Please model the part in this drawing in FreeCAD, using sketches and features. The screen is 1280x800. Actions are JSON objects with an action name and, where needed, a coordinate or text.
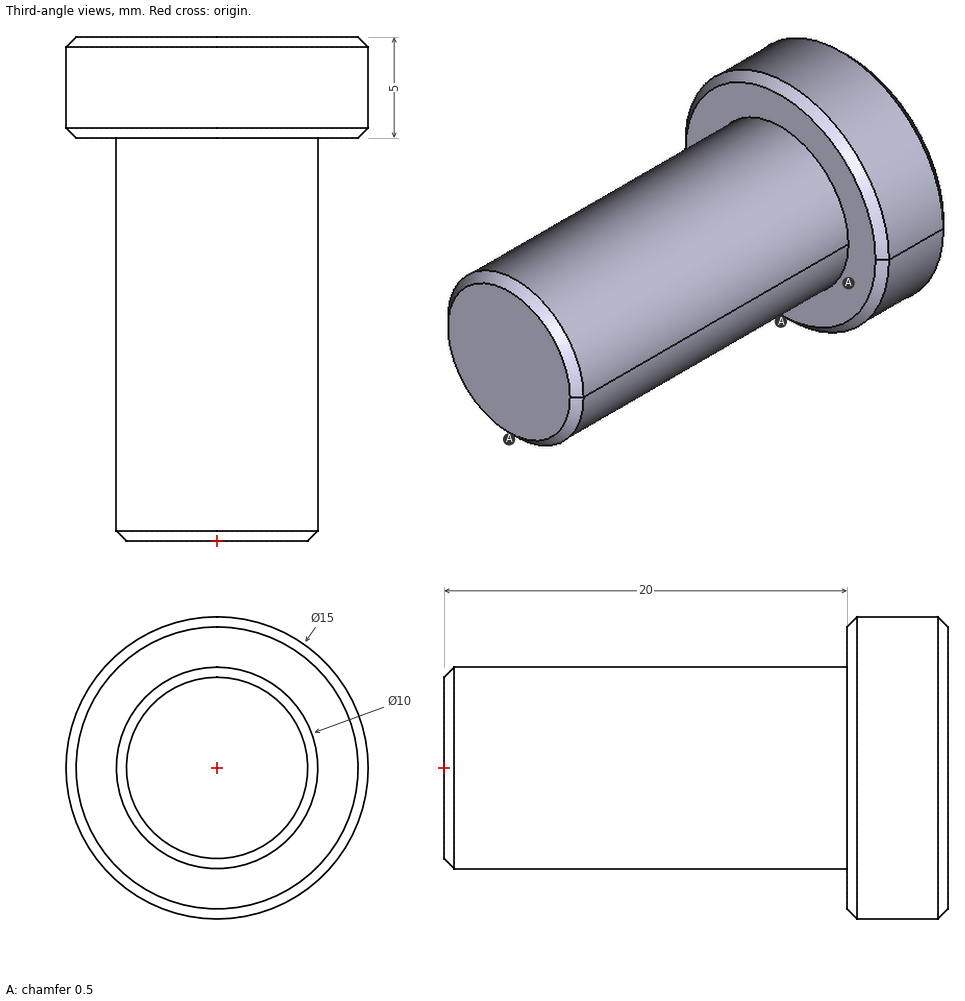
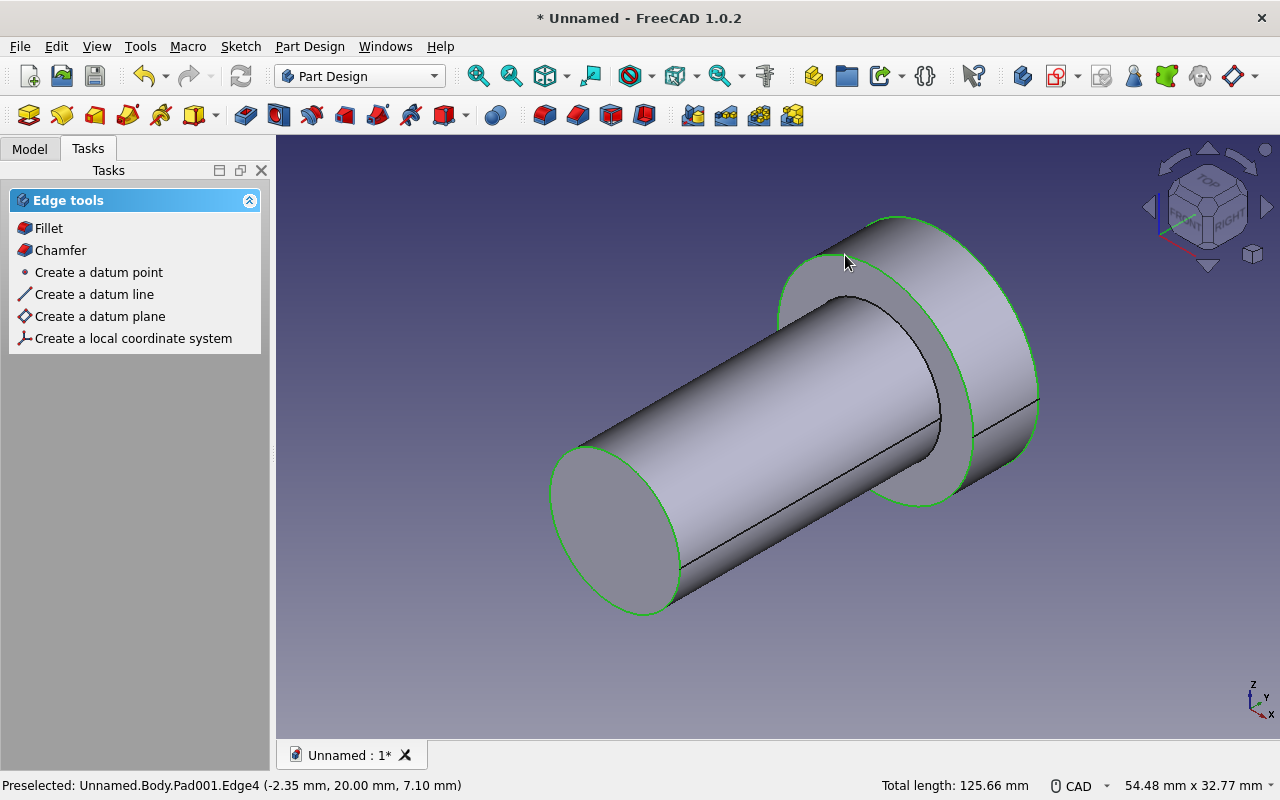
{"action": "left_click", "coordinate": [578, 116]}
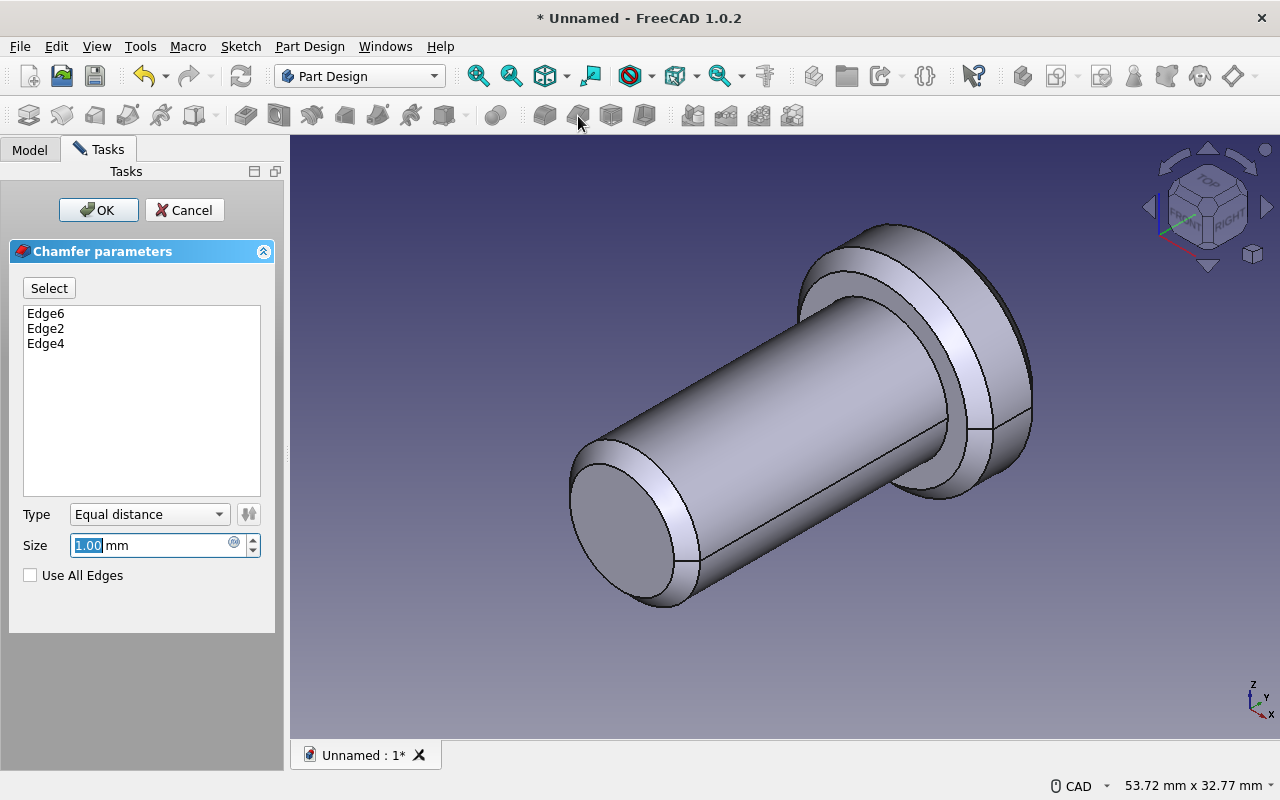
{"action": "type", "text": "0.5"}
{"action": "key", "text": "Tab"}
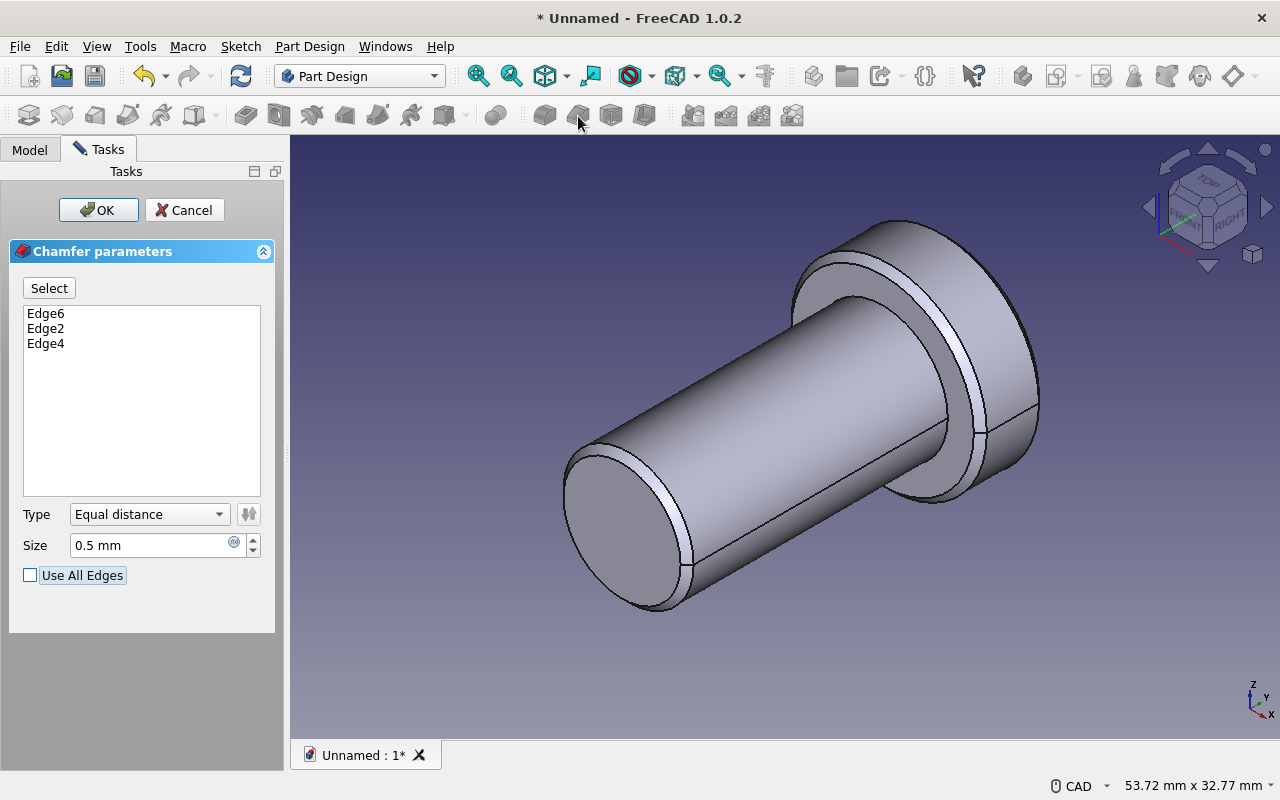
{"action": "left_click", "coordinate": [99, 210]}